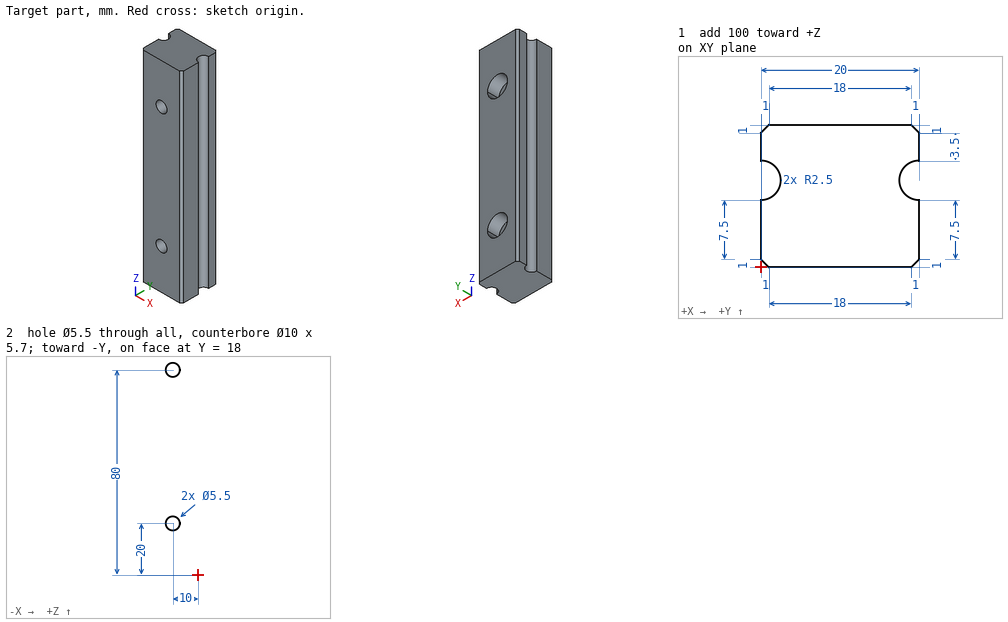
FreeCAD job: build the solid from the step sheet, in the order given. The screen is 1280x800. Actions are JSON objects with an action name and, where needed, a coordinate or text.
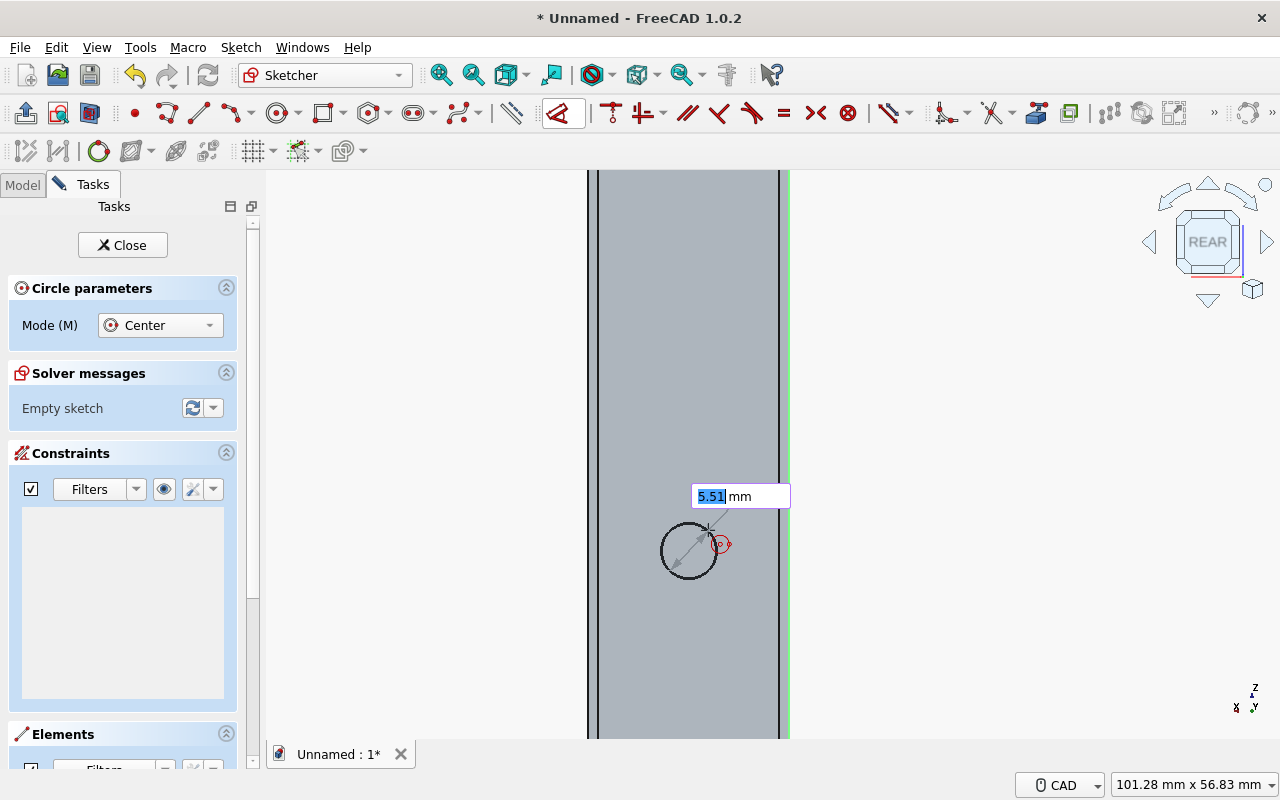
{"action": "type", "text": "5.5"}
{"action": "key", "text": "Return"}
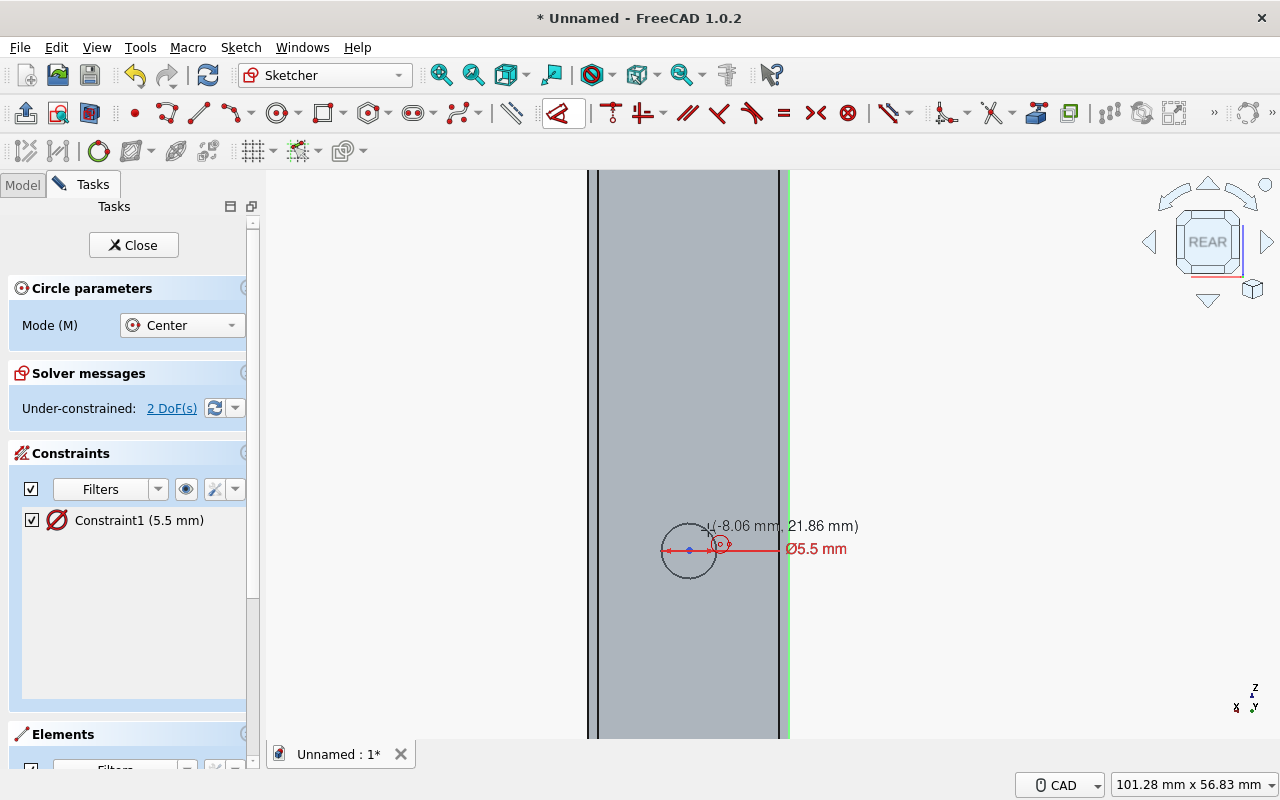
{"action": "scroll", "coordinate": [688, 552], "scroll_direction": "down", "scroll_amount": 4}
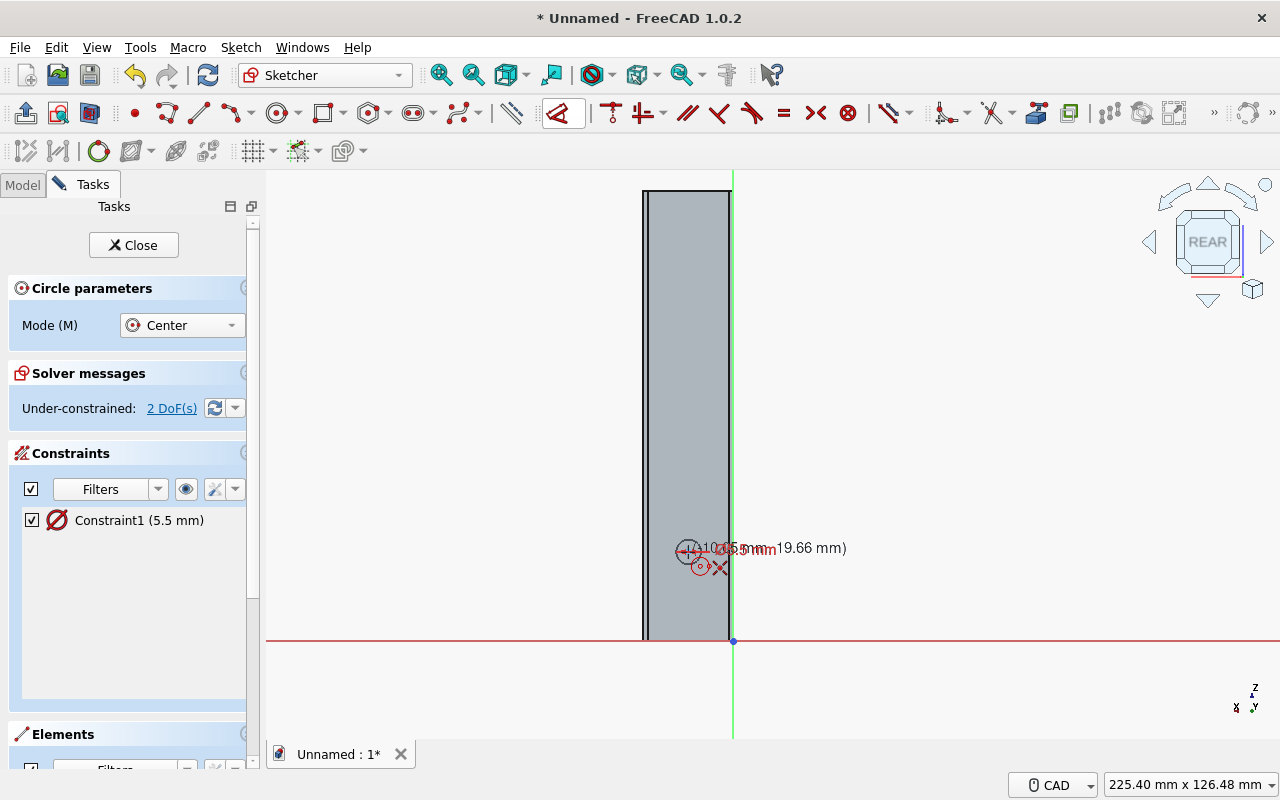
{"action": "scroll", "coordinate": [688, 281], "scroll_direction": "up", "scroll_amount": 4}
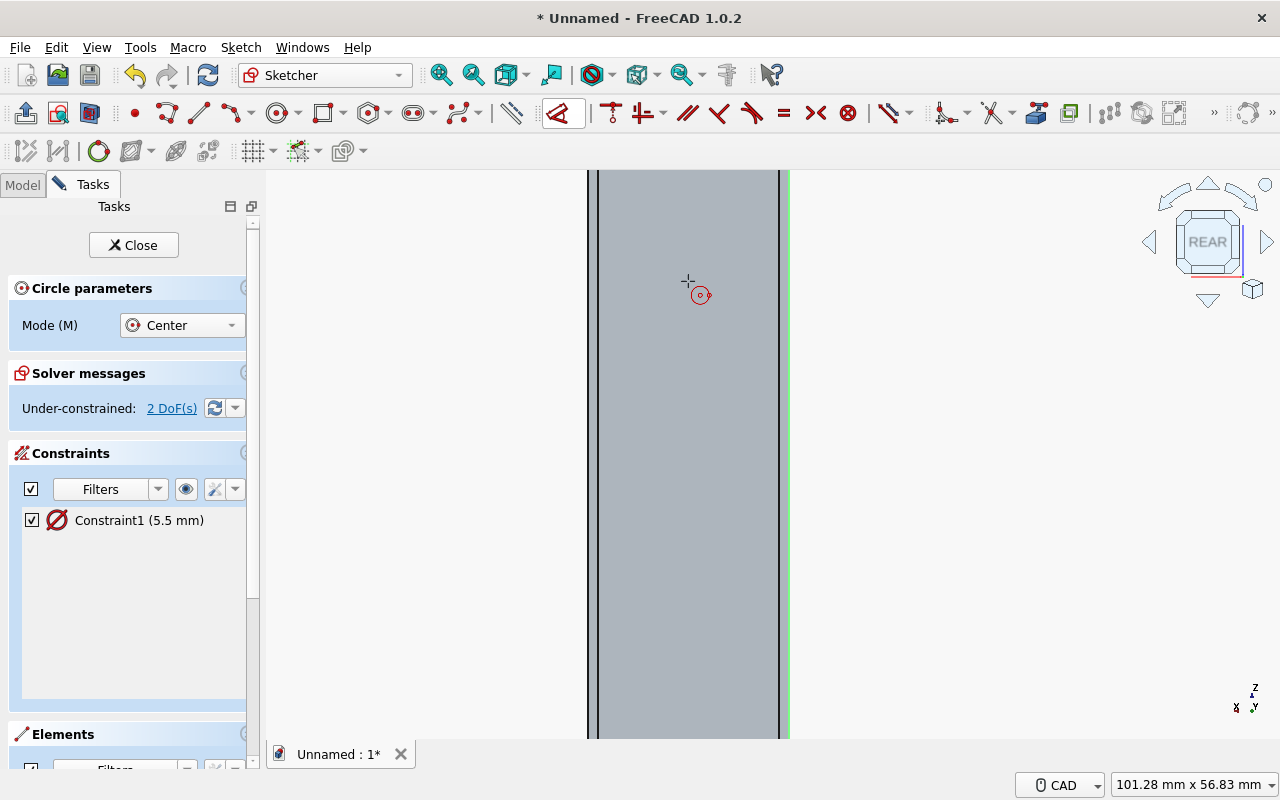
{"action": "left_click", "coordinate": [689, 282]}
{"action": "mouse_move", "coordinate": [708, 262]}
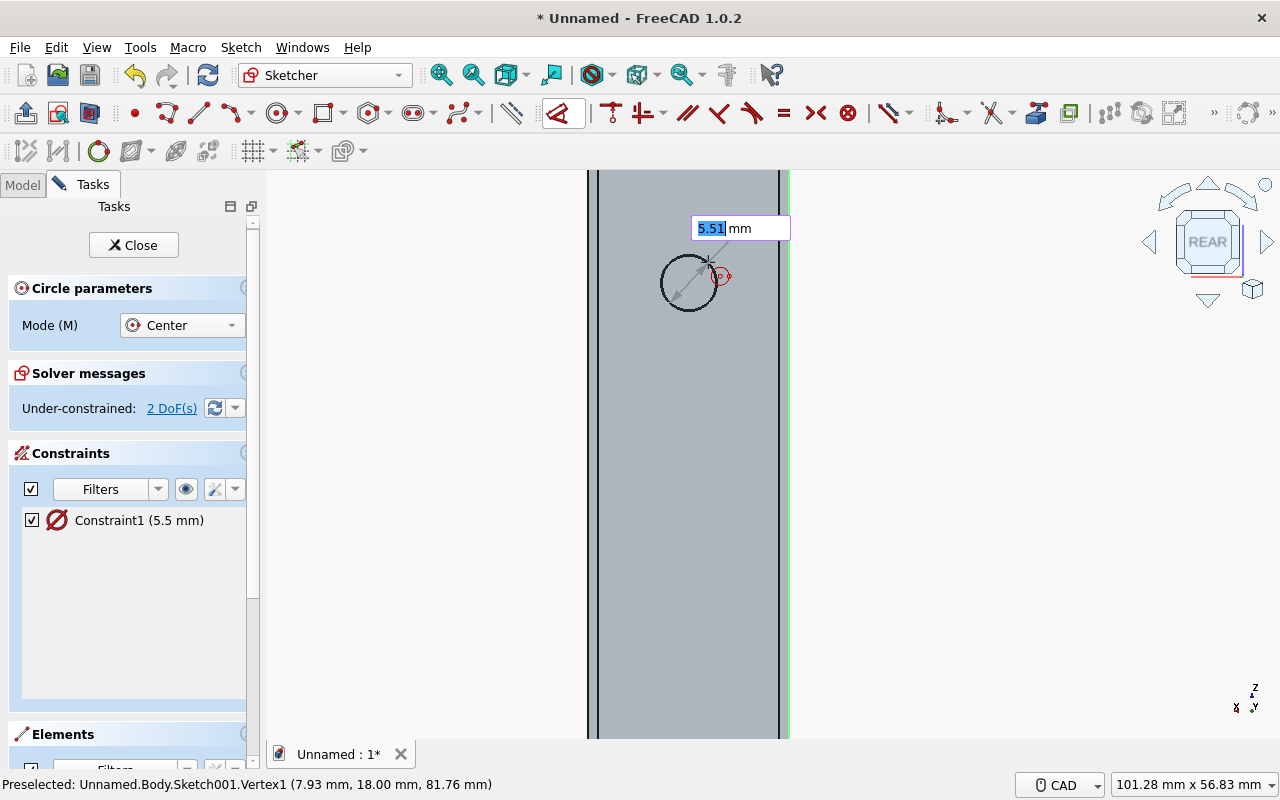
{"action": "type", "text": "5.5"}
{"action": "key", "text": "Return"}
{"action": "key", "text": "Escape"}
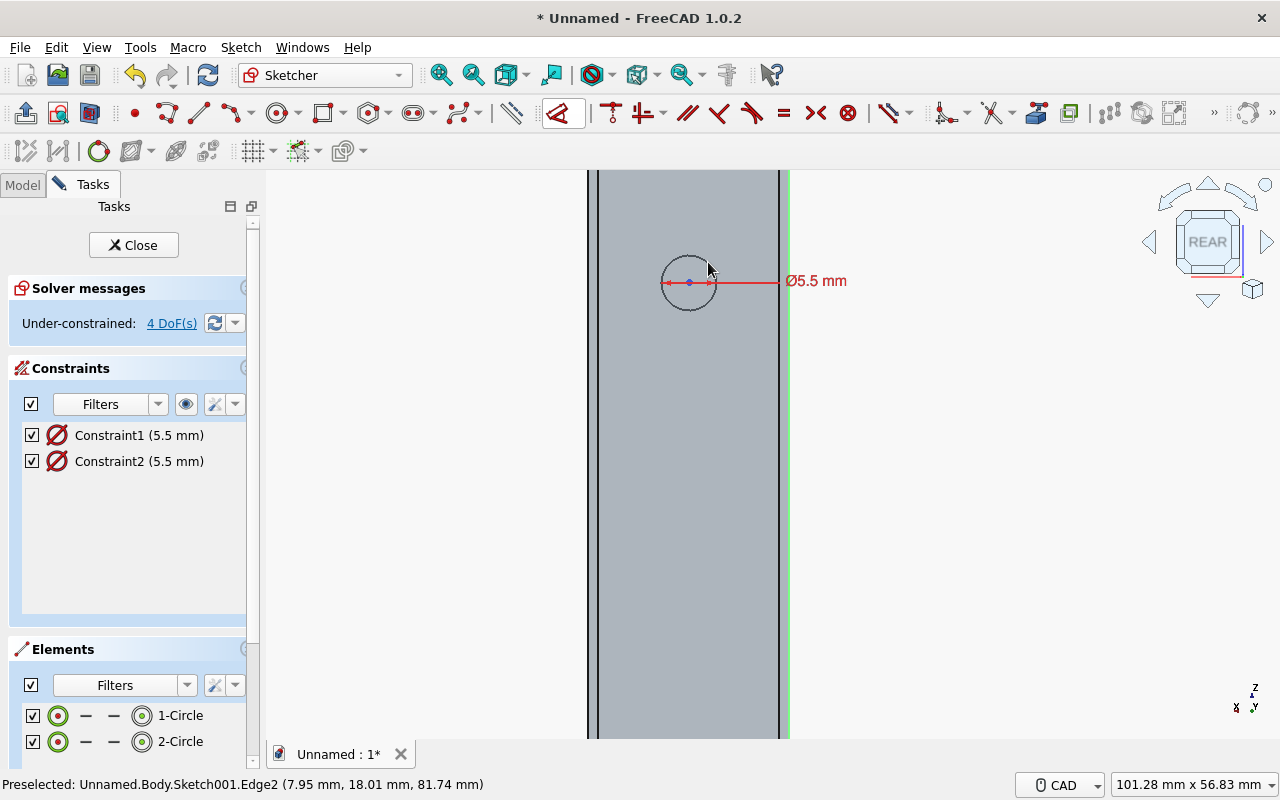
{"action": "scroll", "coordinate": [688, 280], "scroll_direction": "down", "scroll_amount": 4}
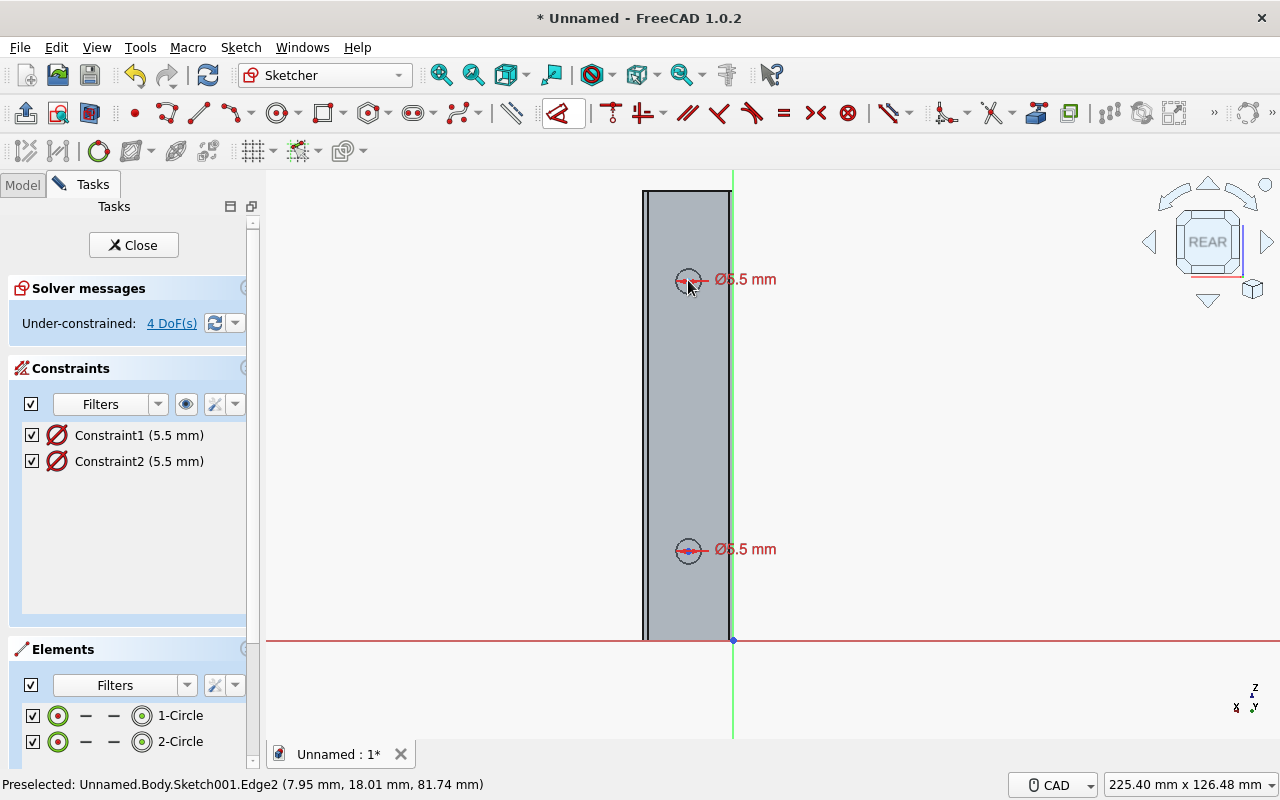
{"action": "left_click", "coordinate": [689, 551]}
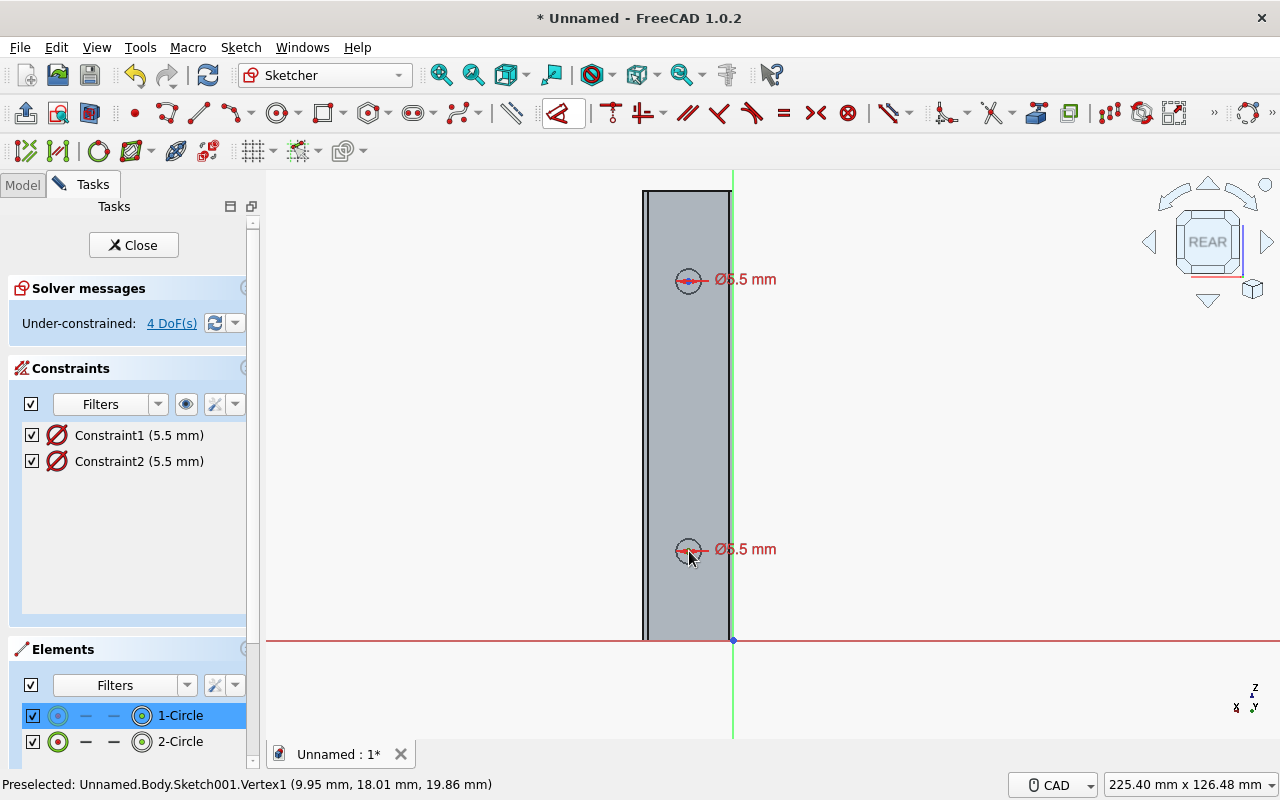
{"action": "left_click", "coordinate": [689, 281]}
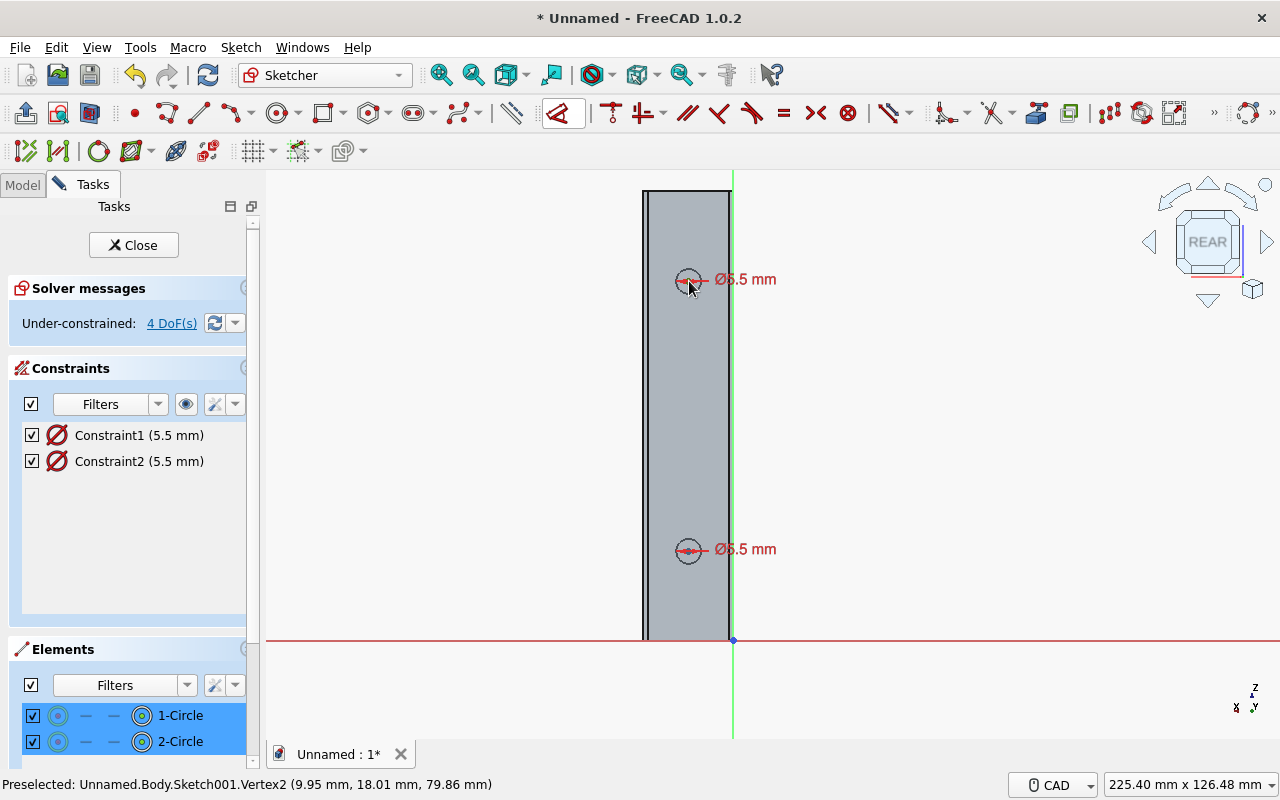
{"action": "key", "text": "v"}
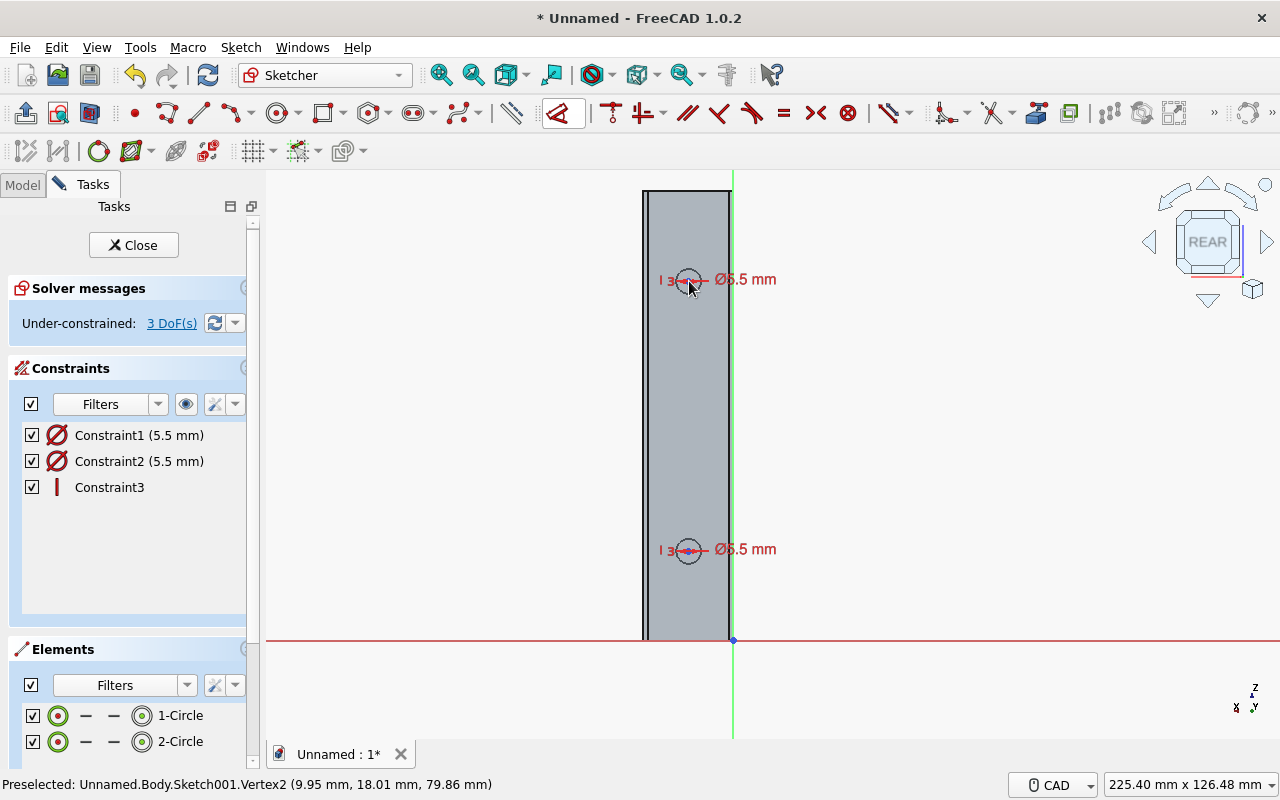
{"action": "left_click", "coordinate": [689, 551]}